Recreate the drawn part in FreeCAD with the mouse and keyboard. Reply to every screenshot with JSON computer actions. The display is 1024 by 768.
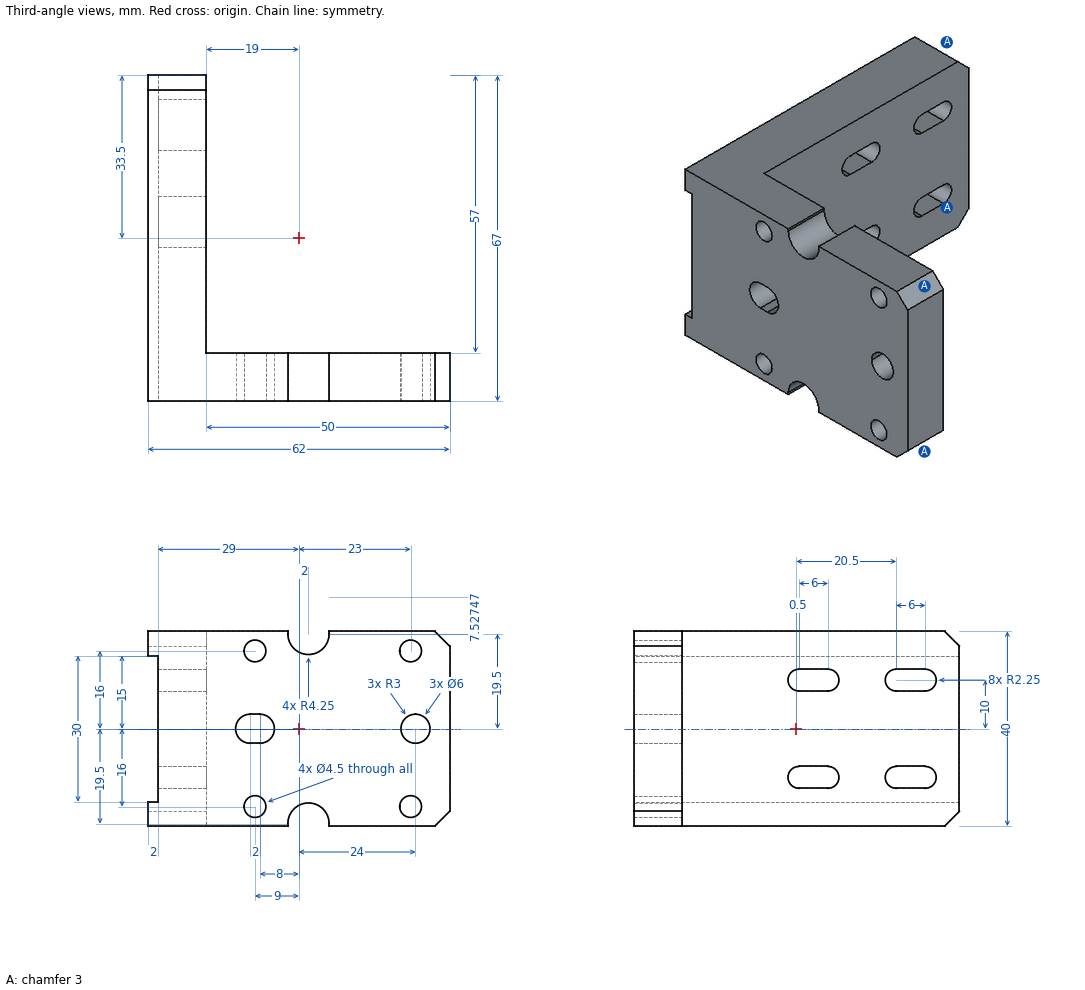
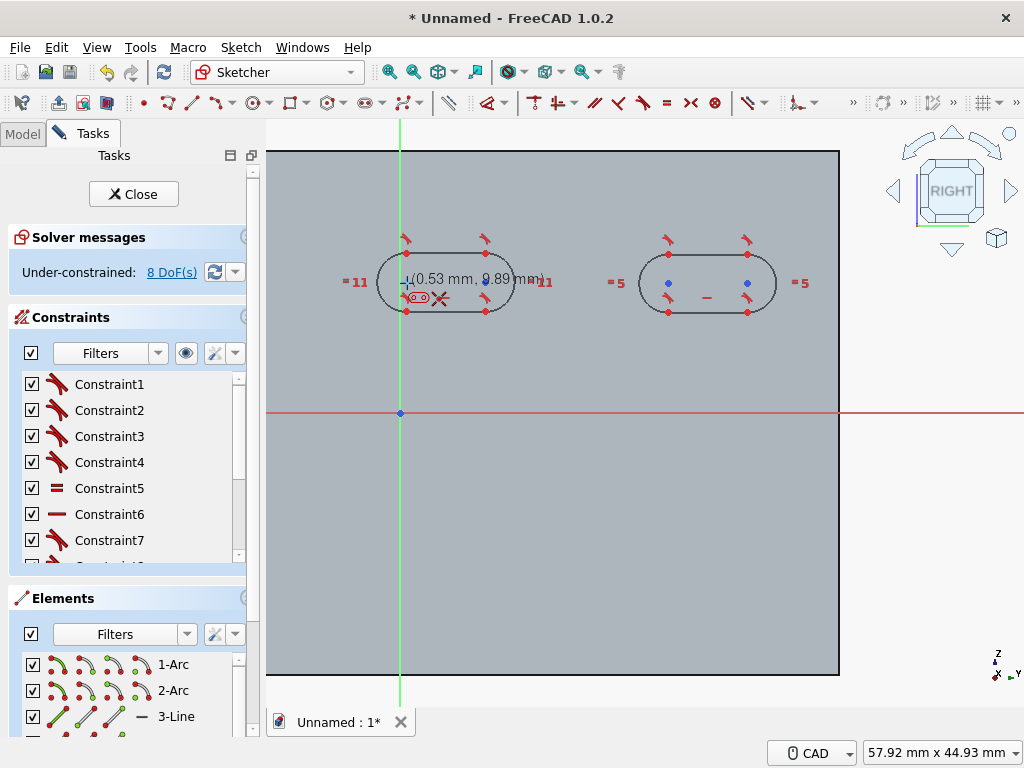
{"action": "left_click", "coordinate": [668, 544]}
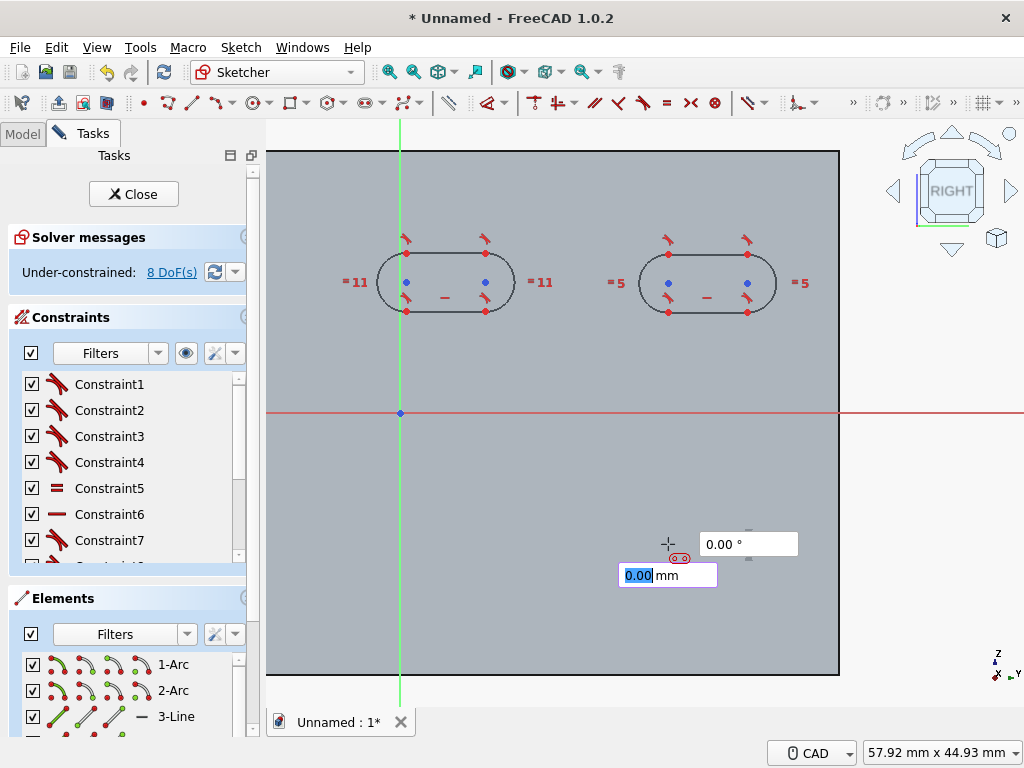
{"action": "left_click", "coordinate": [747, 544]}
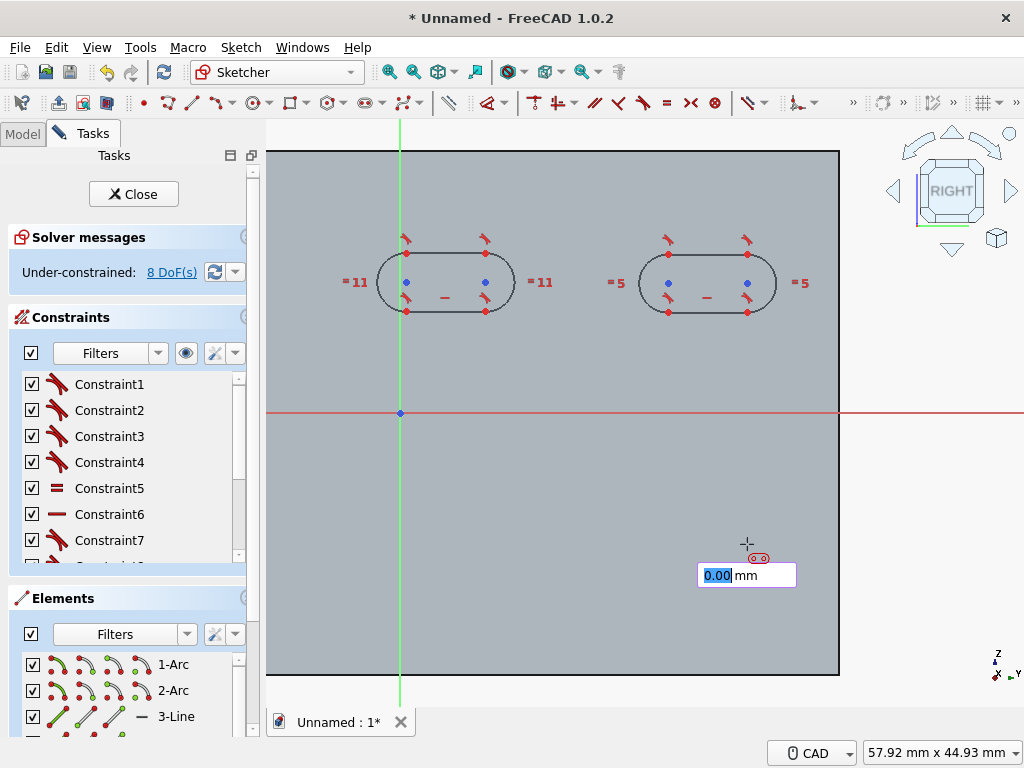
{"action": "left_click", "coordinate": [708, 573]}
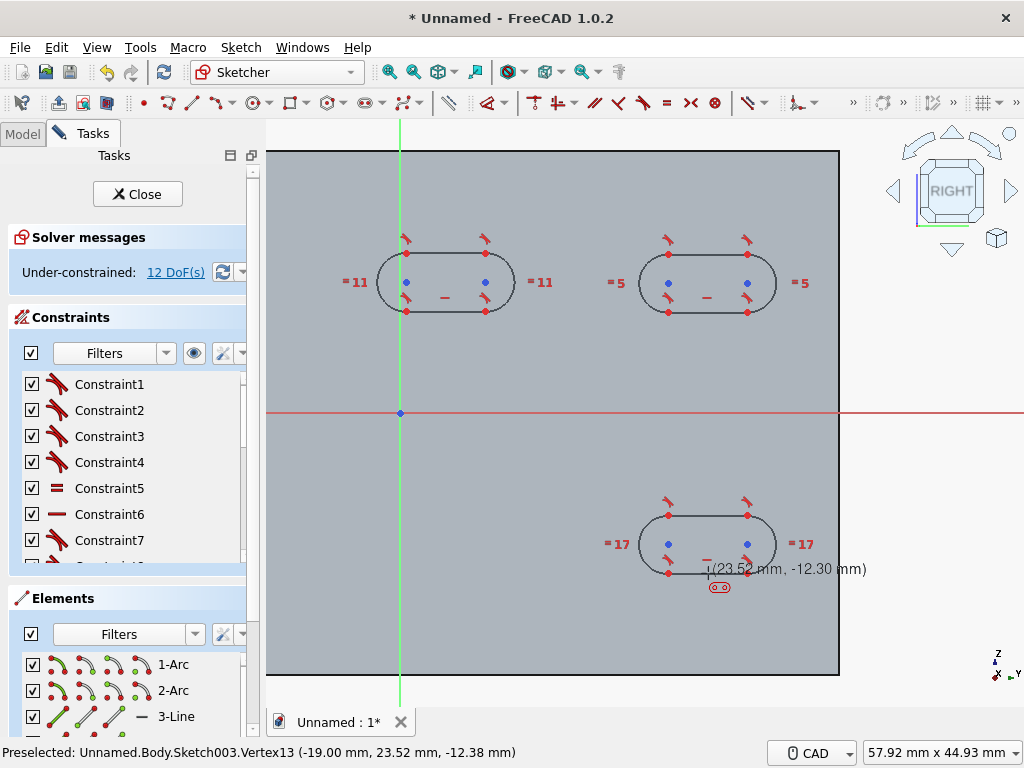
{"action": "scroll", "coordinate": [407, 544], "scroll_direction": "up", "scroll_amount": 5}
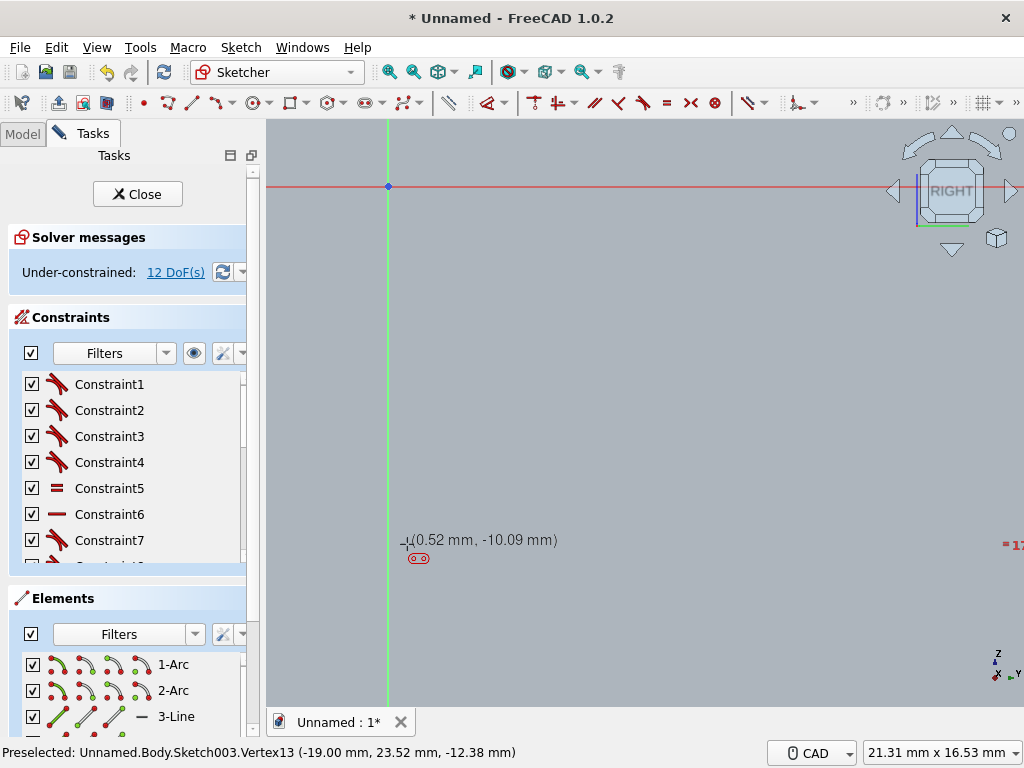
{"action": "left_click", "coordinate": [406, 542]}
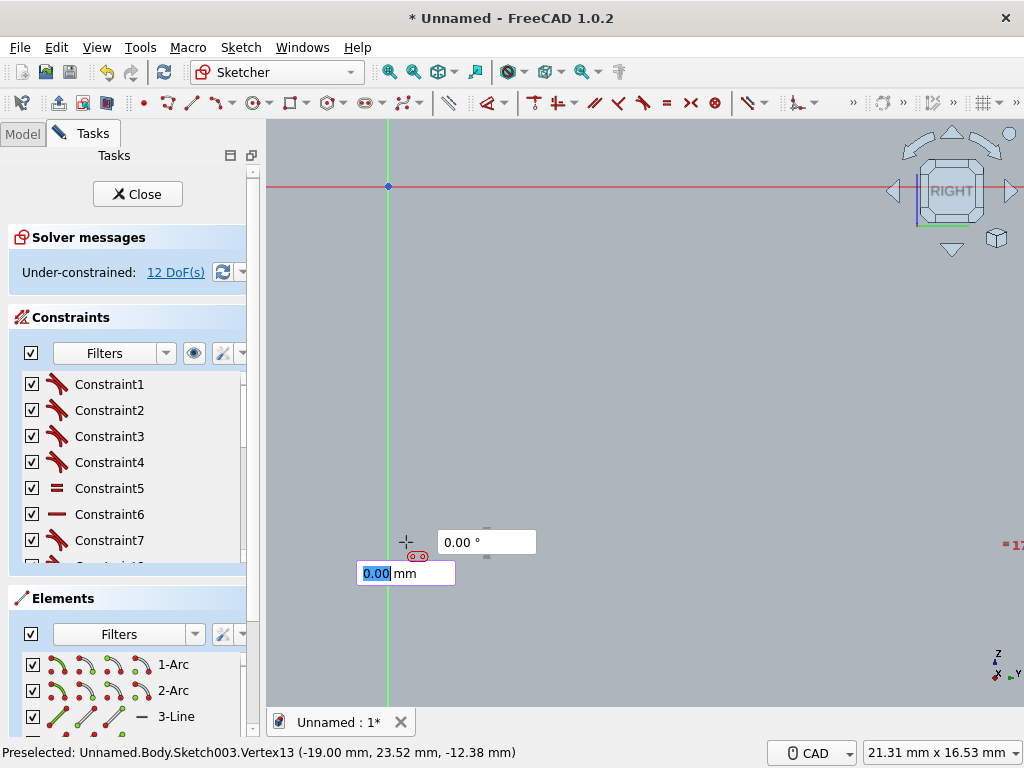
{"action": "left_click", "coordinate": [619, 542]}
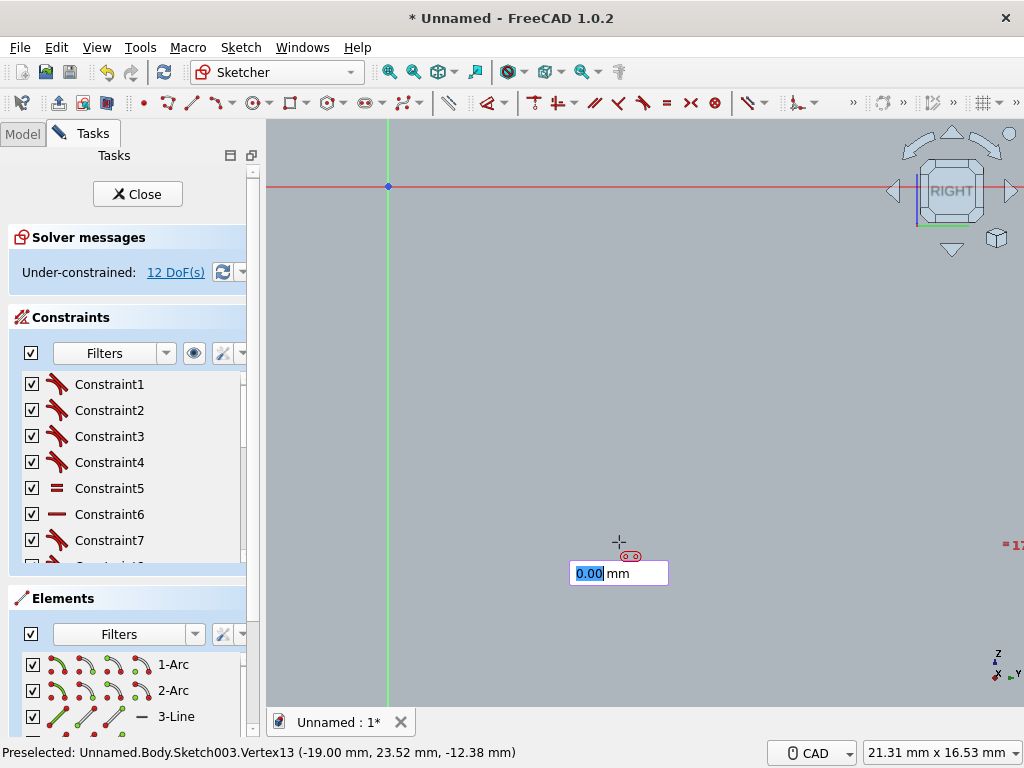
{"action": "left_click", "coordinate": [513, 622]}
{"action": "key", "text": "Escape"}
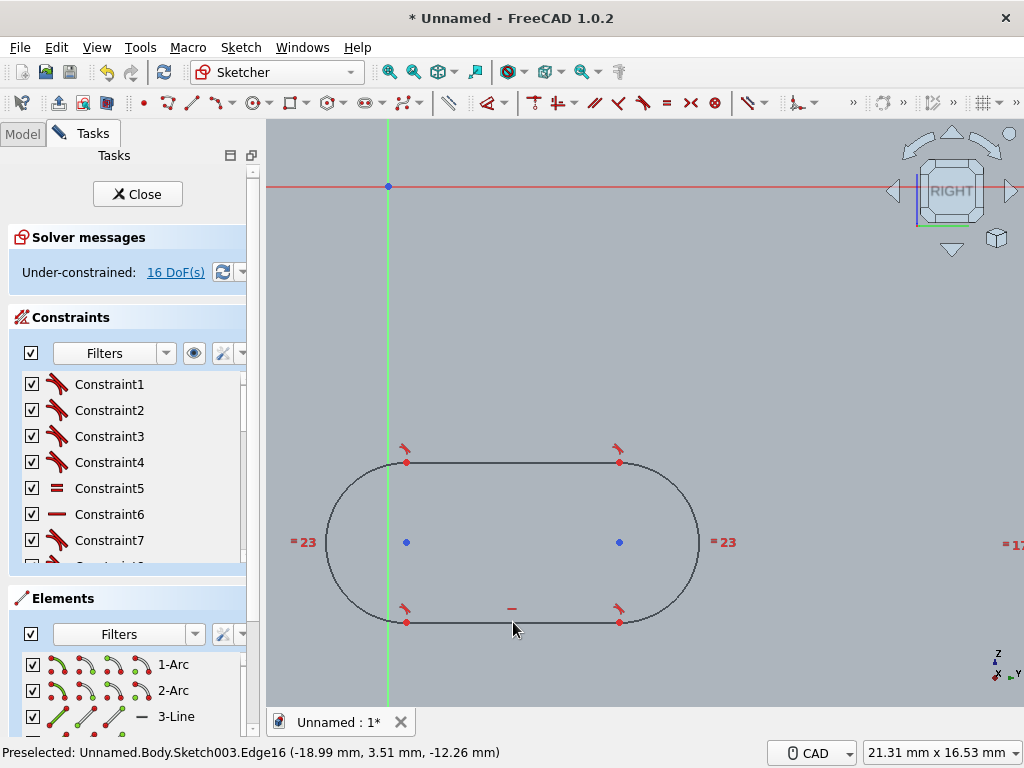
{"action": "scroll", "coordinate": [407, 545], "scroll_direction": "down", "scroll_amount": 5}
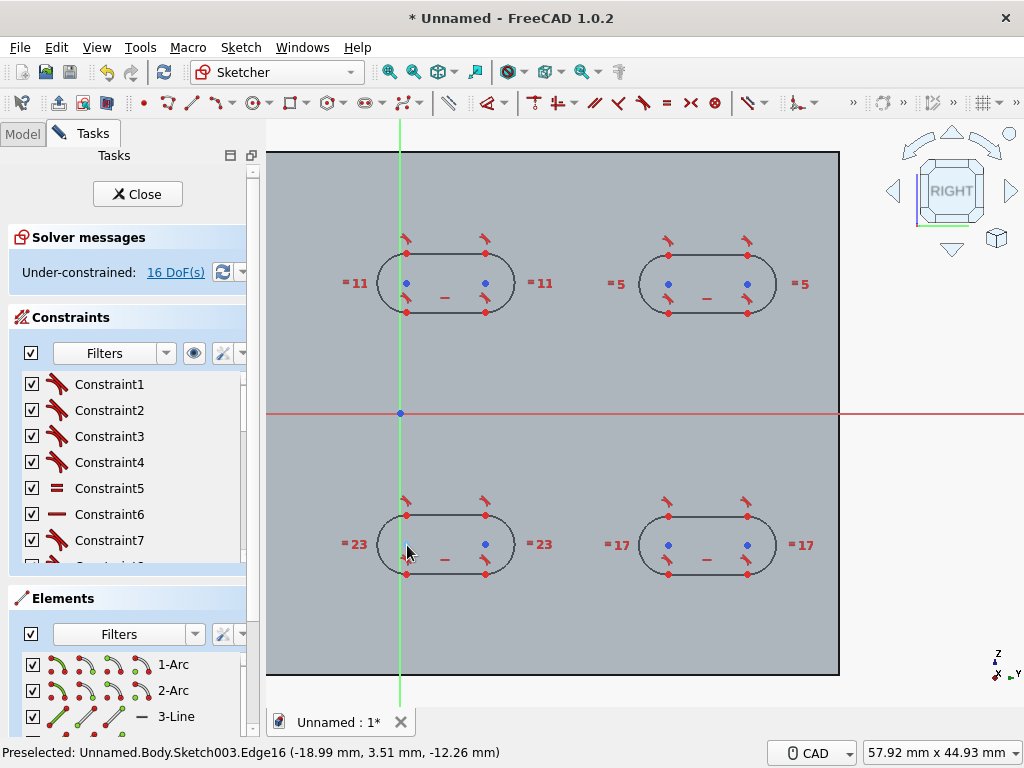
{"action": "left_click", "coordinate": [645, 267]}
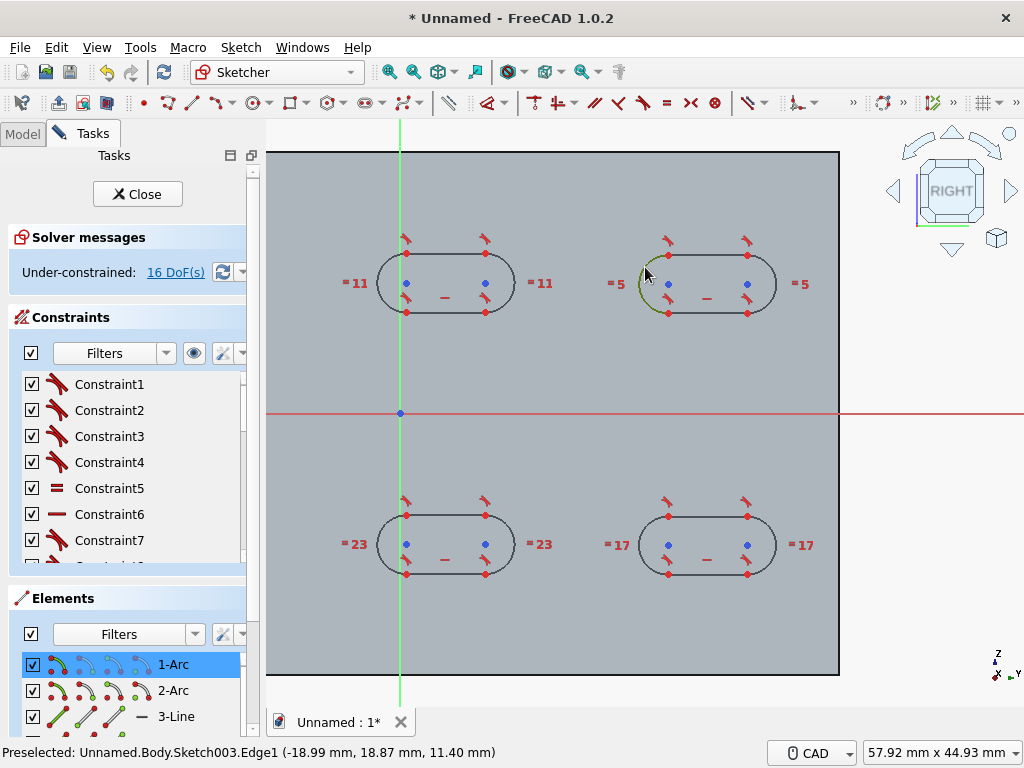
{"action": "left_click", "coordinate": [383, 266]}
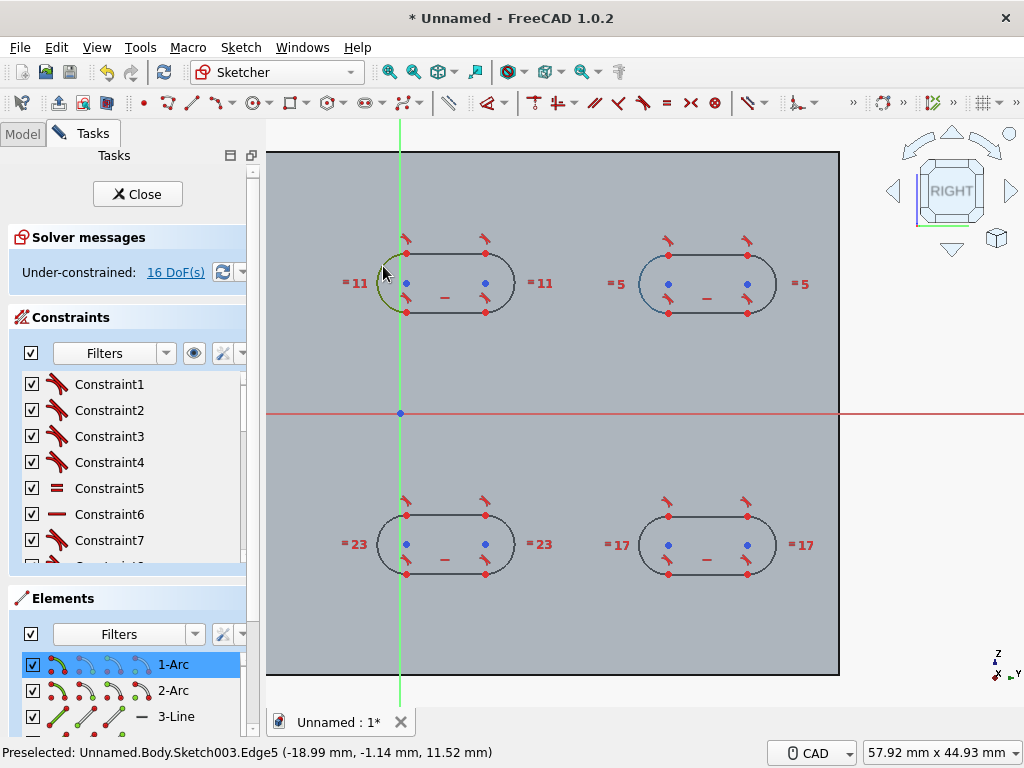
{"action": "left_click", "coordinate": [645, 529]}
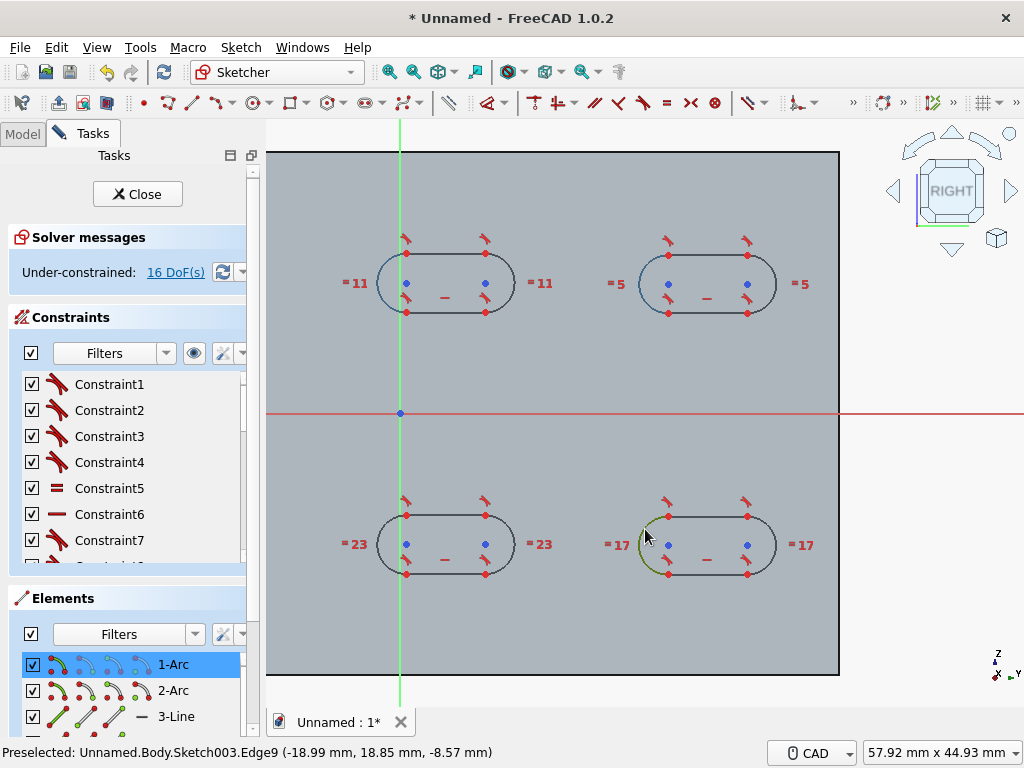
{"action": "left_click", "coordinate": [383, 527]}